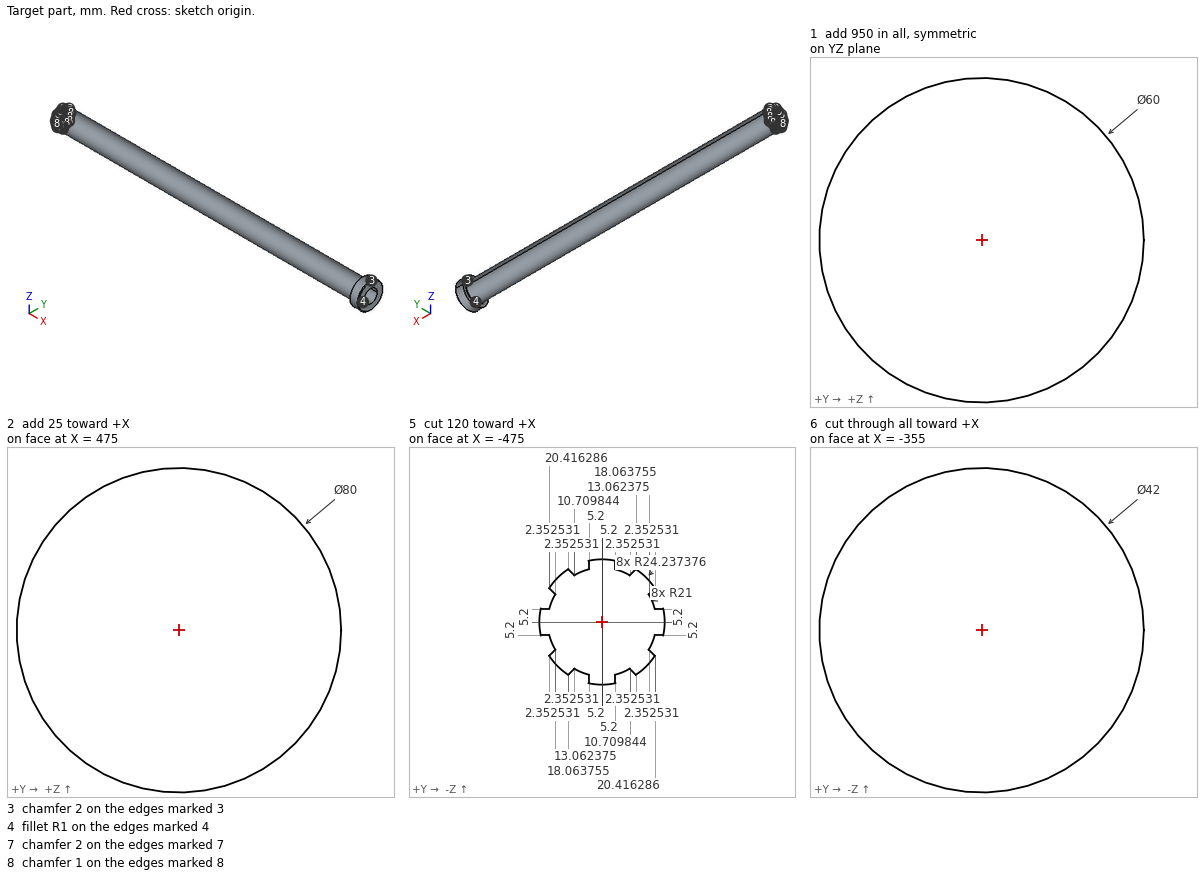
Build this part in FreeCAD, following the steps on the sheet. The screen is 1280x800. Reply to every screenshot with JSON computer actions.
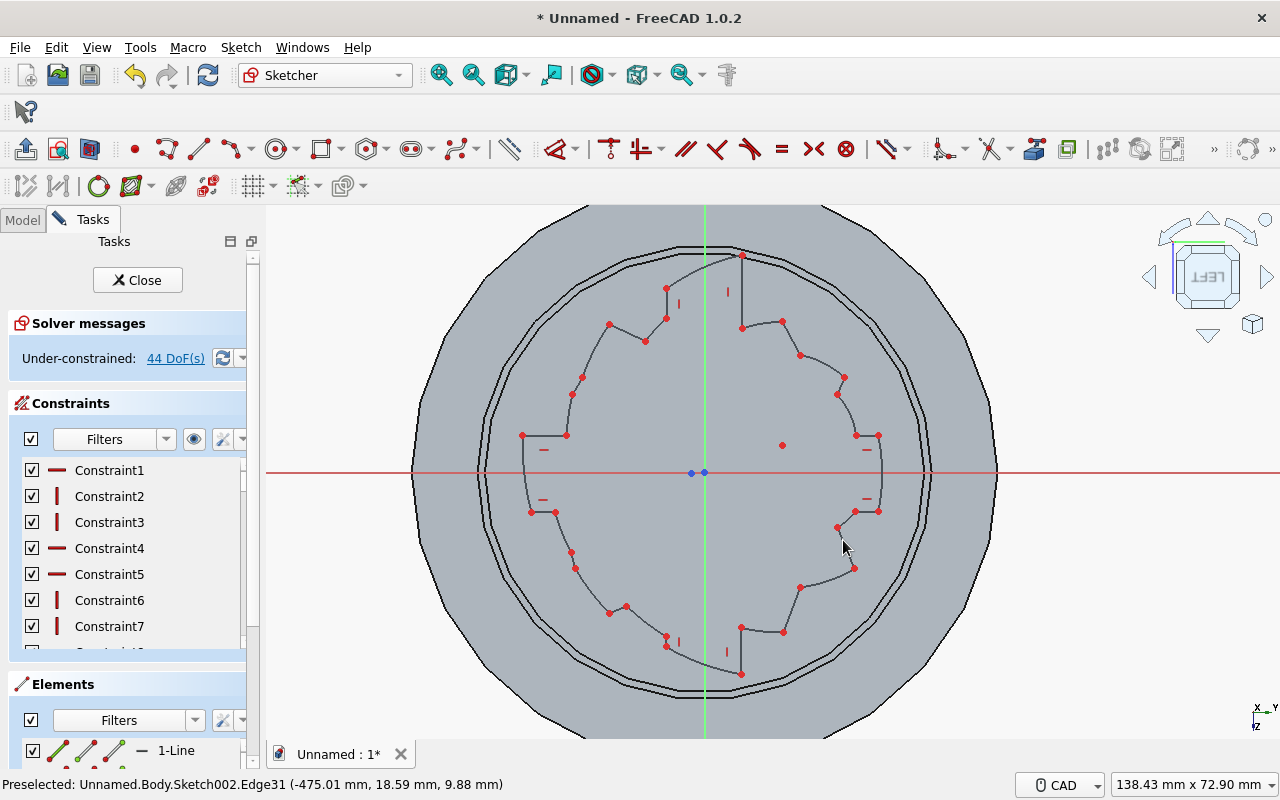
{"action": "left_click", "coordinate": [853, 422]}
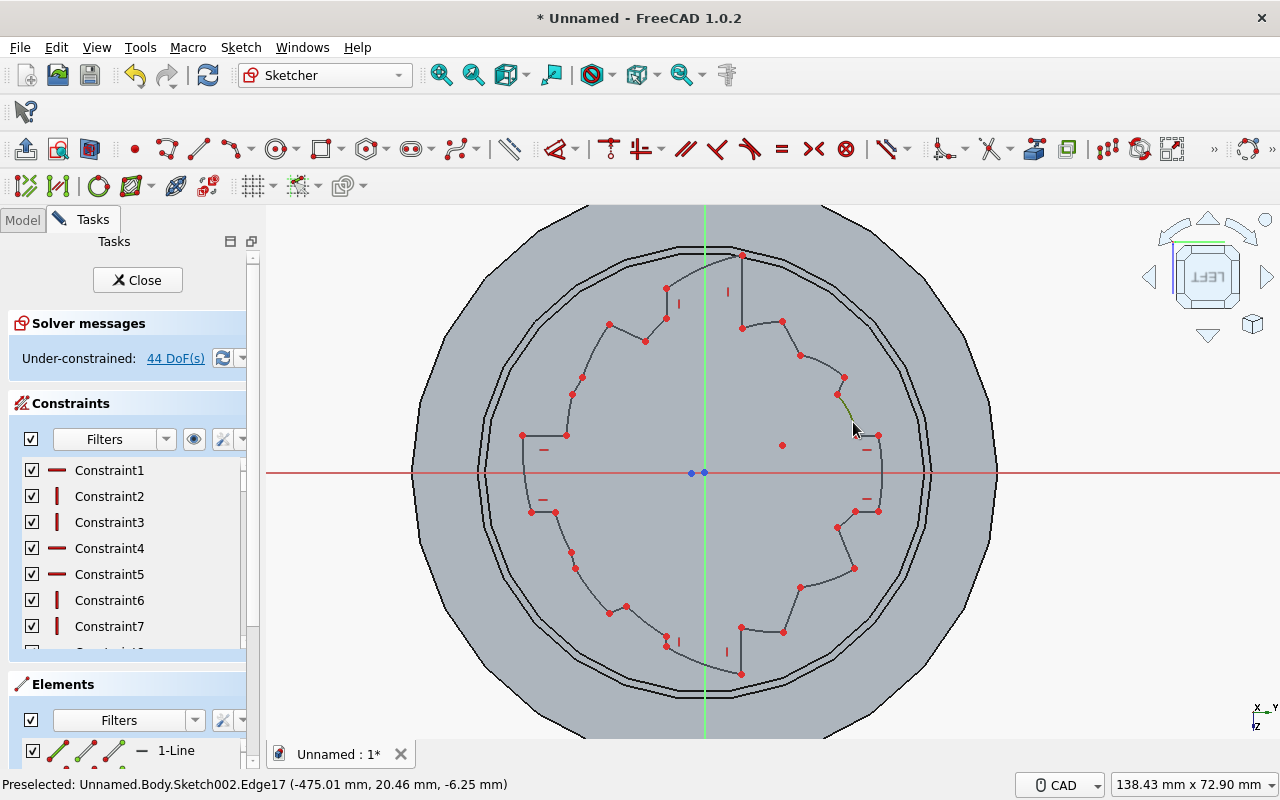
{"action": "left_click", "coordinate": [881, 489]}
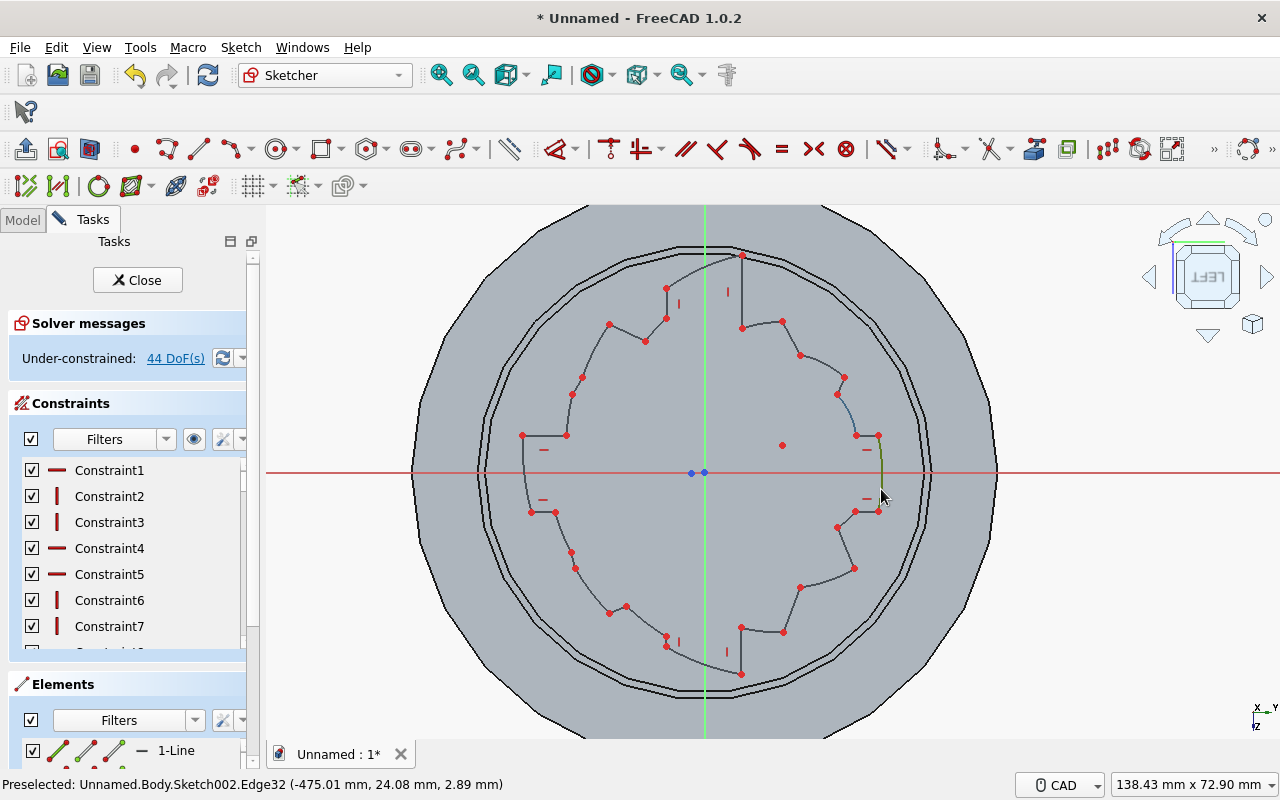
{"action": "key", "text": "c"}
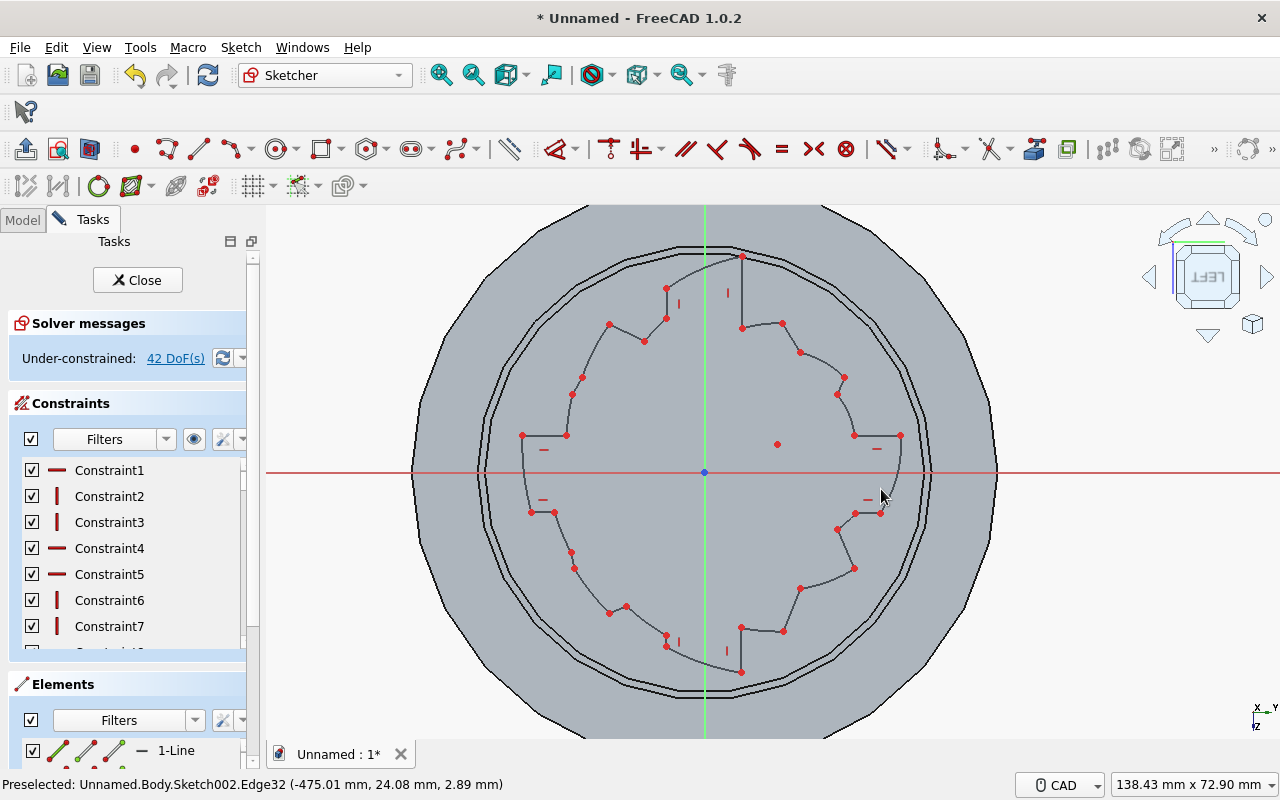
{"action": "left_click_drag", "start_coordinate": [695, 435], "coordinate": [788, 483]}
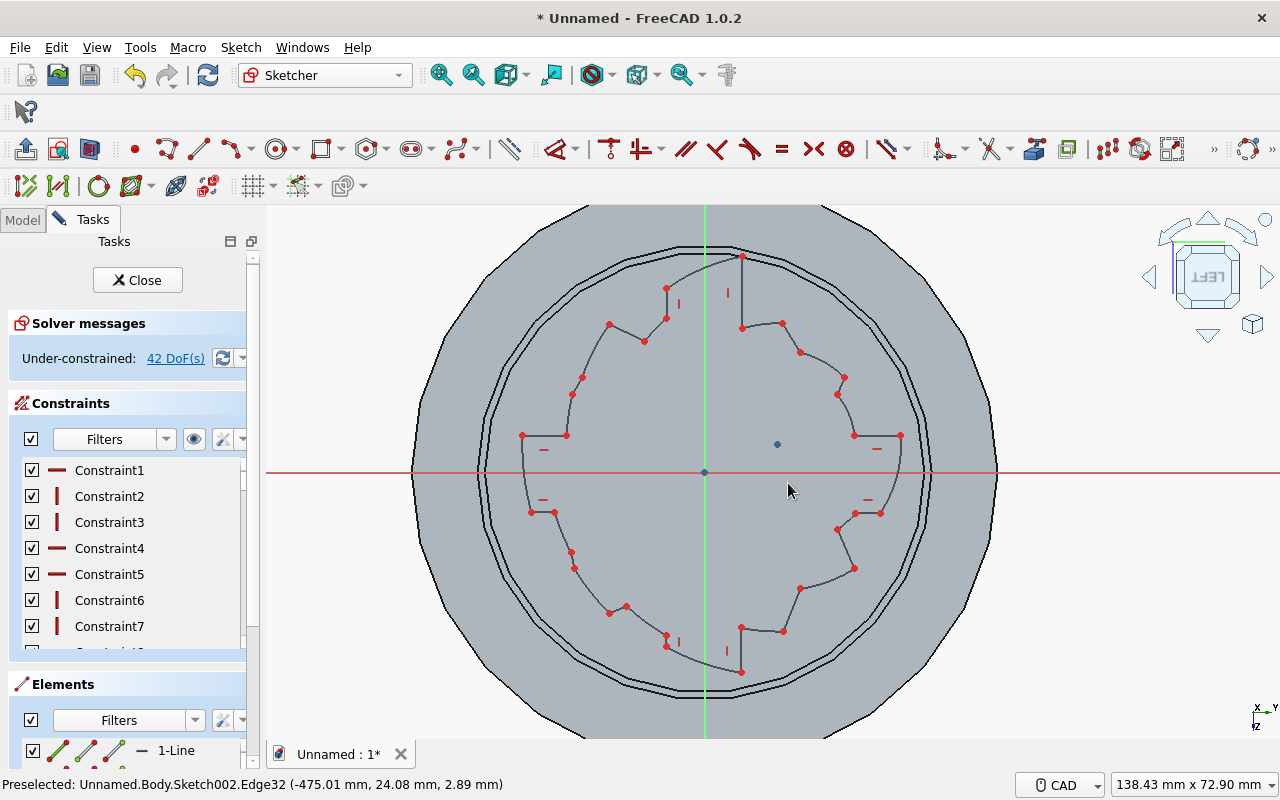
{"action": "left_click", "coordinate": [610, 150]}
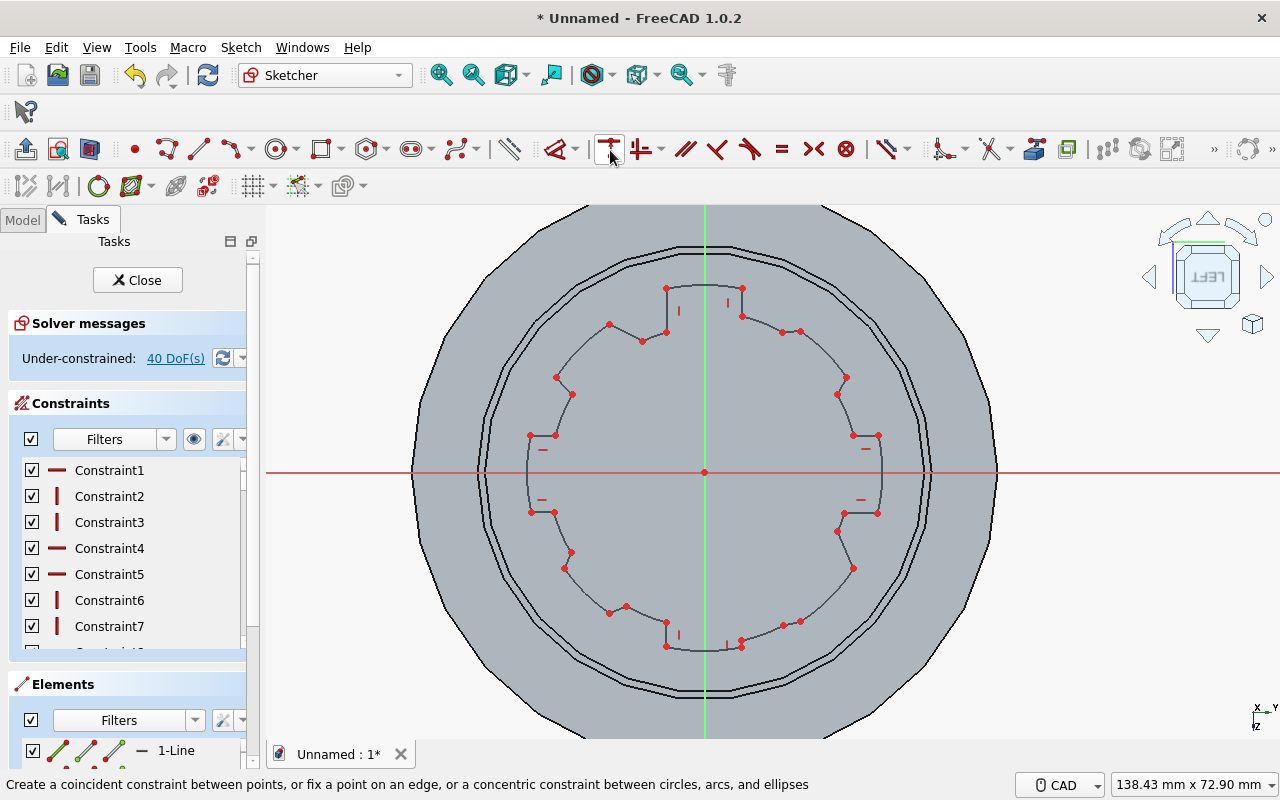
{"action": "left_click", "coordinate": [850, 423]}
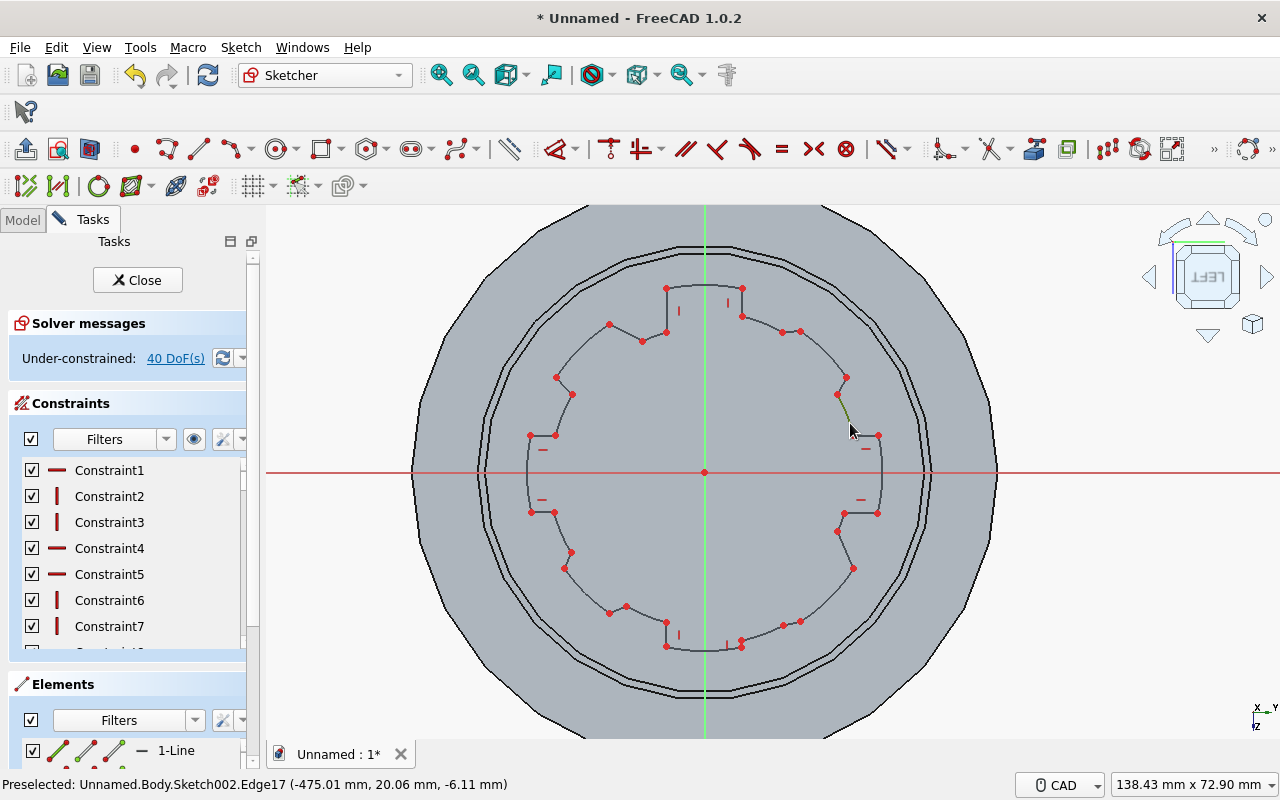
{"action": "left_click", "coordinate": [771, 326]}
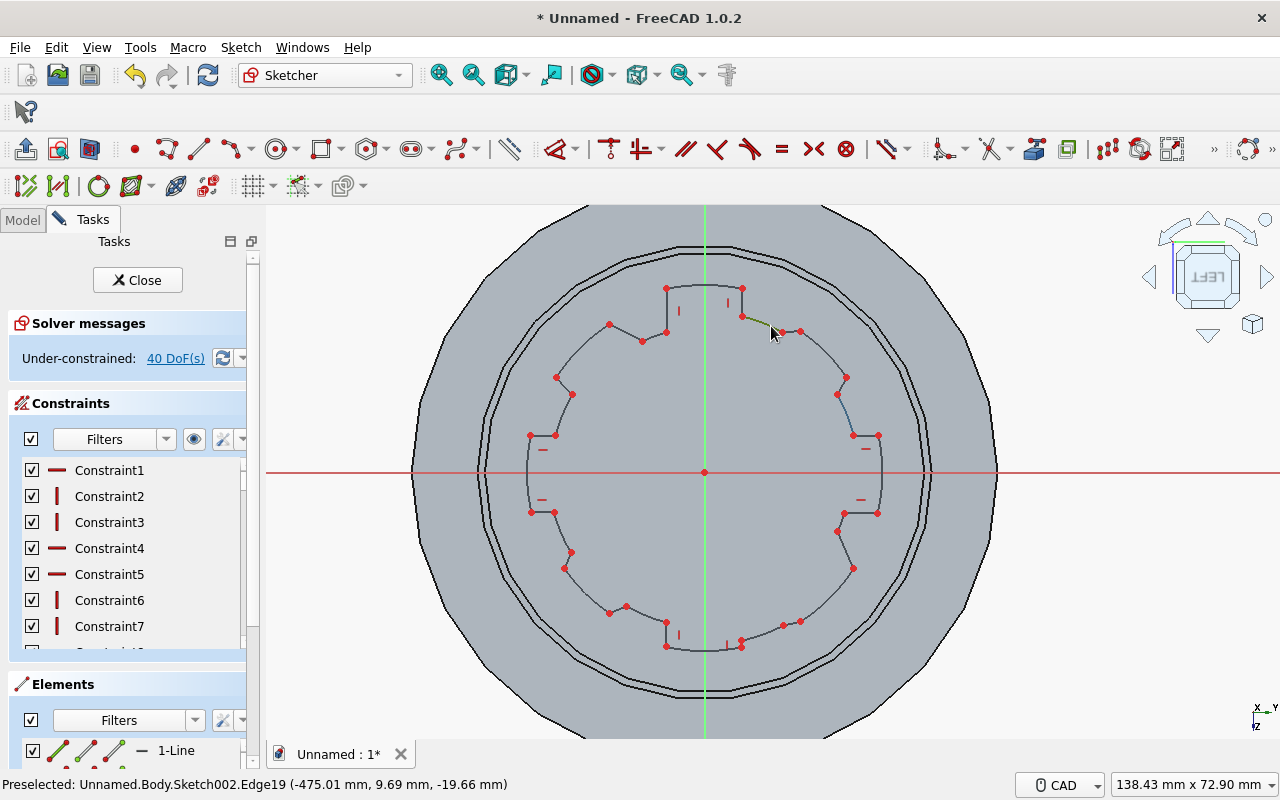
{"action": "left_click", "coordinate": [655, 336]}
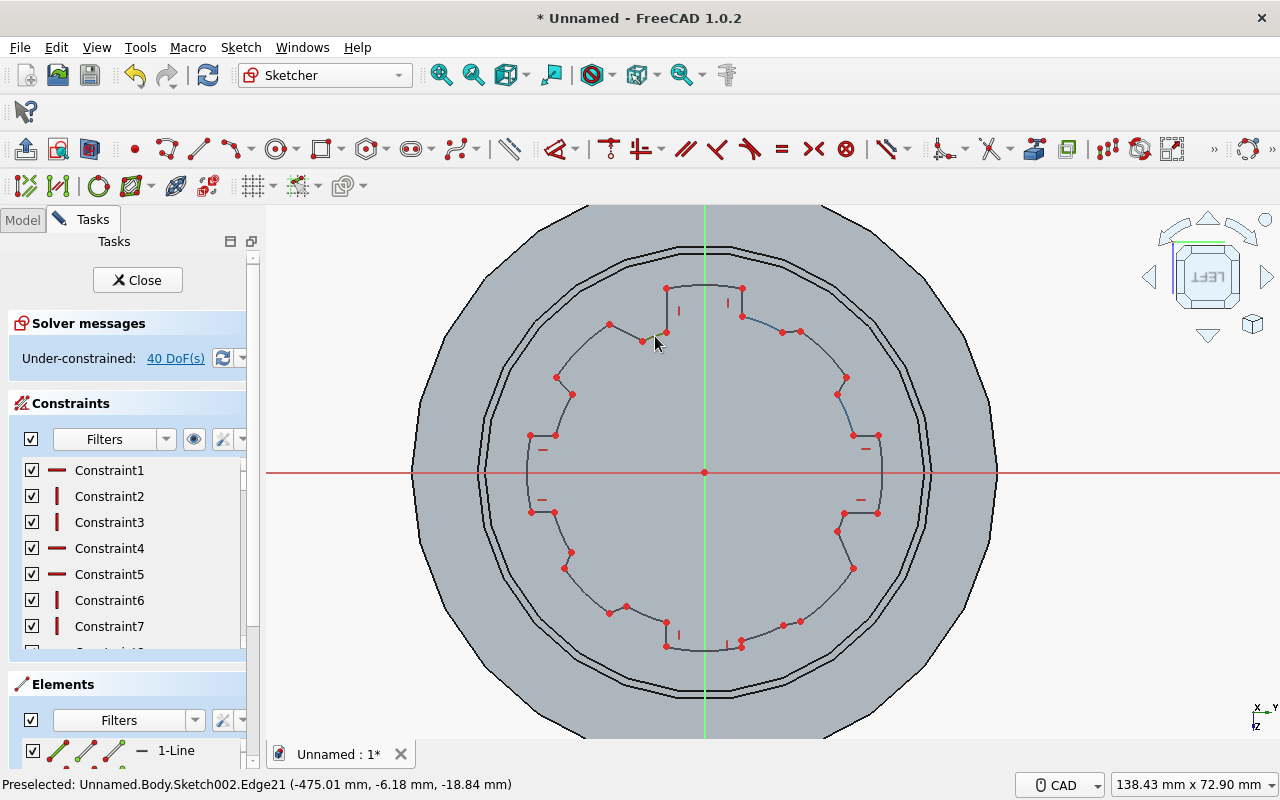
{"action": "left_click", "coordinate": [566, 407]}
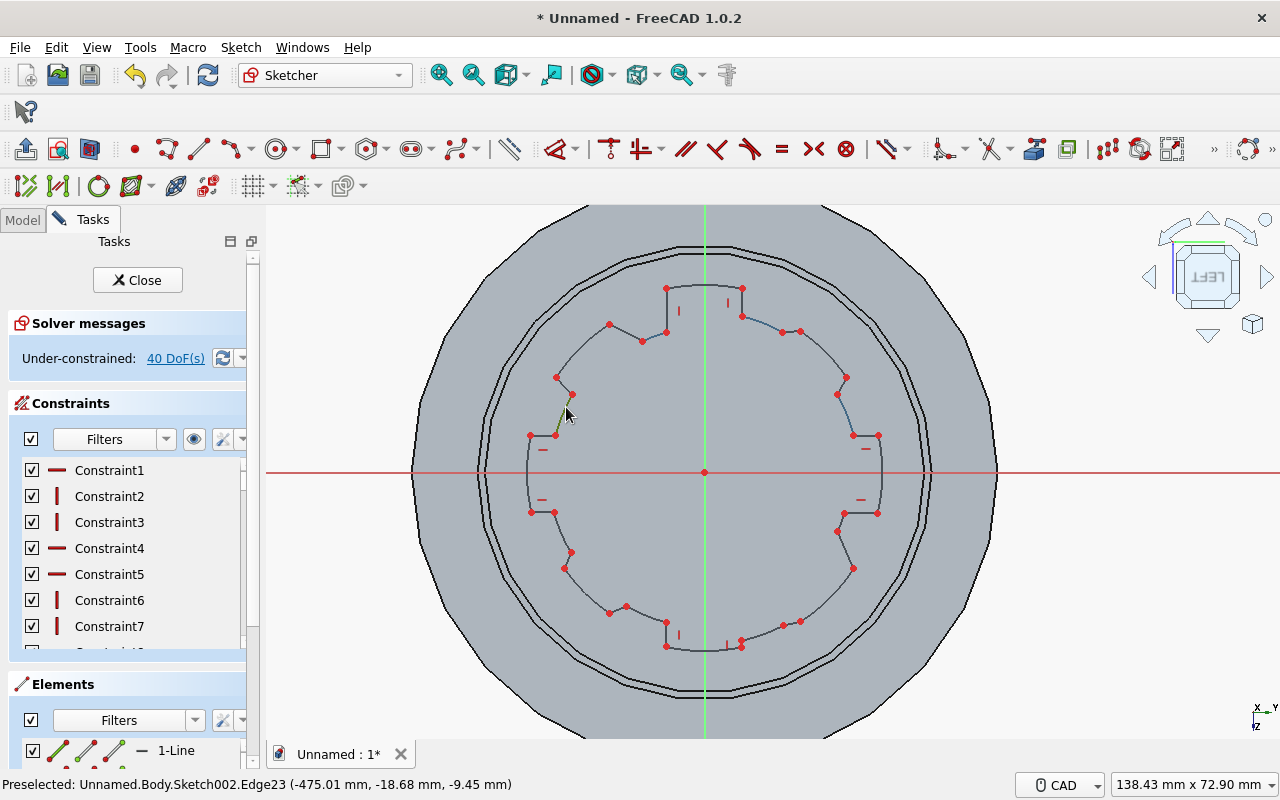
{"action": "left_click", "coordinate": [558, 525]}